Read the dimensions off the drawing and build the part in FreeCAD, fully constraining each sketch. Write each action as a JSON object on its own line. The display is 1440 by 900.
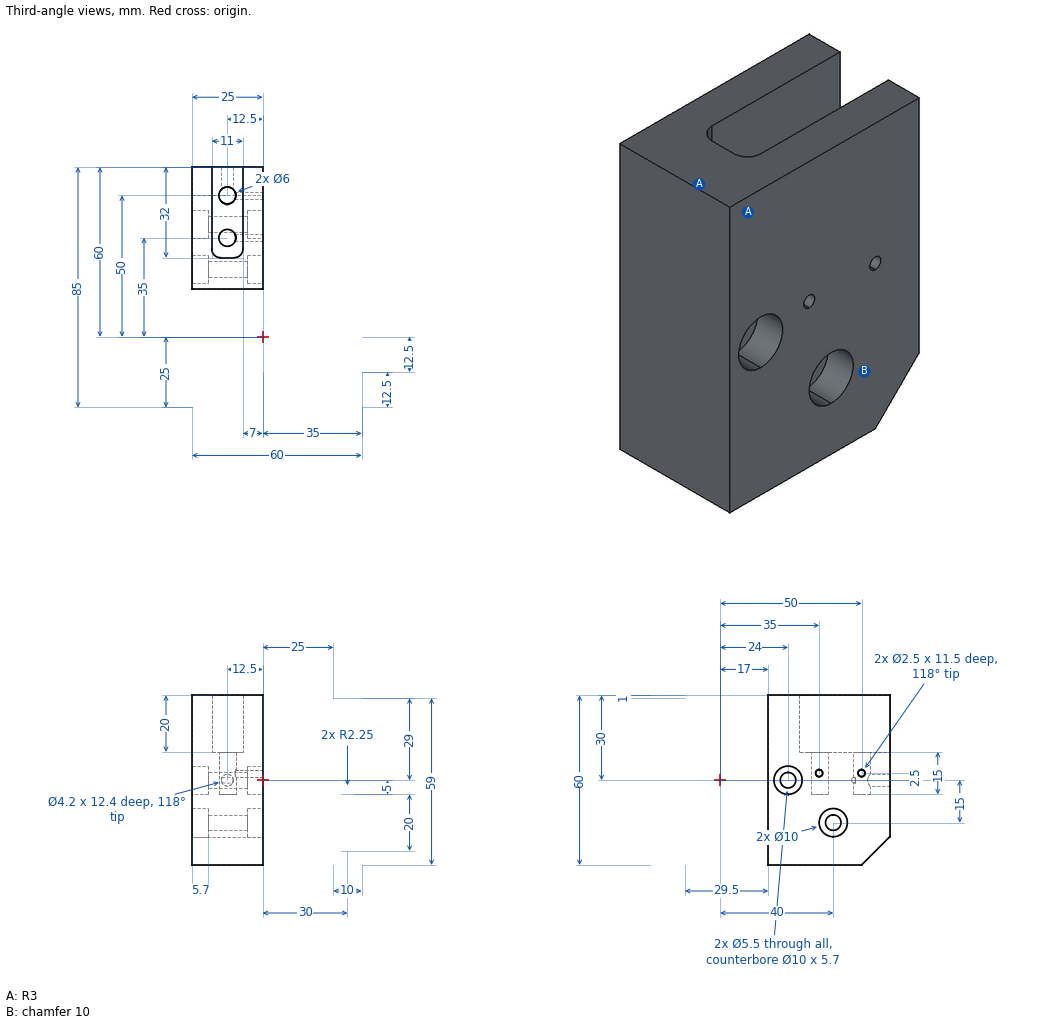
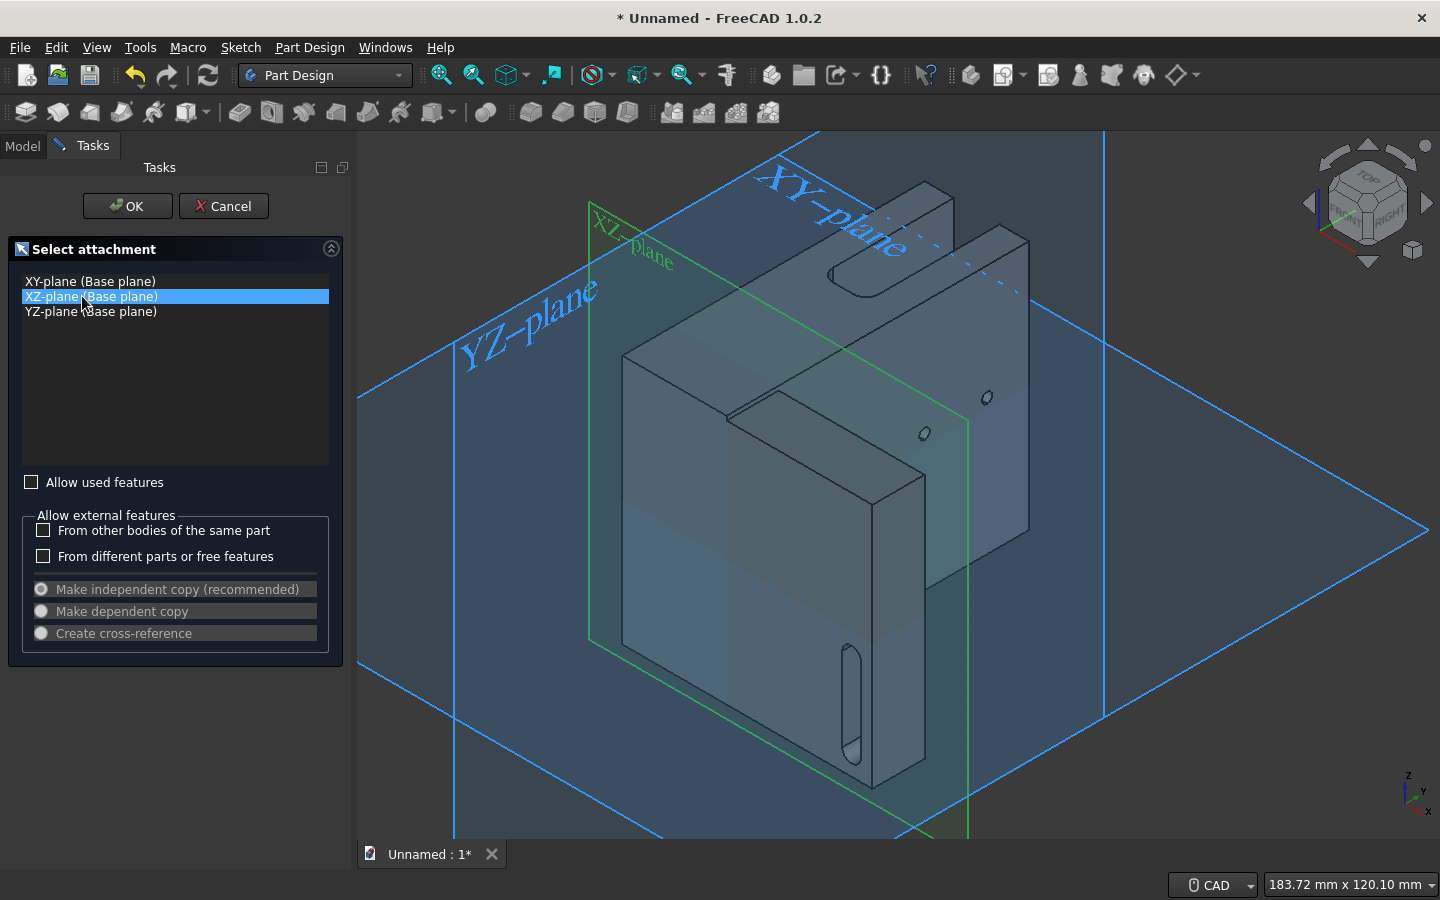
{"action": "left_click", "coordinate": [128, 206]}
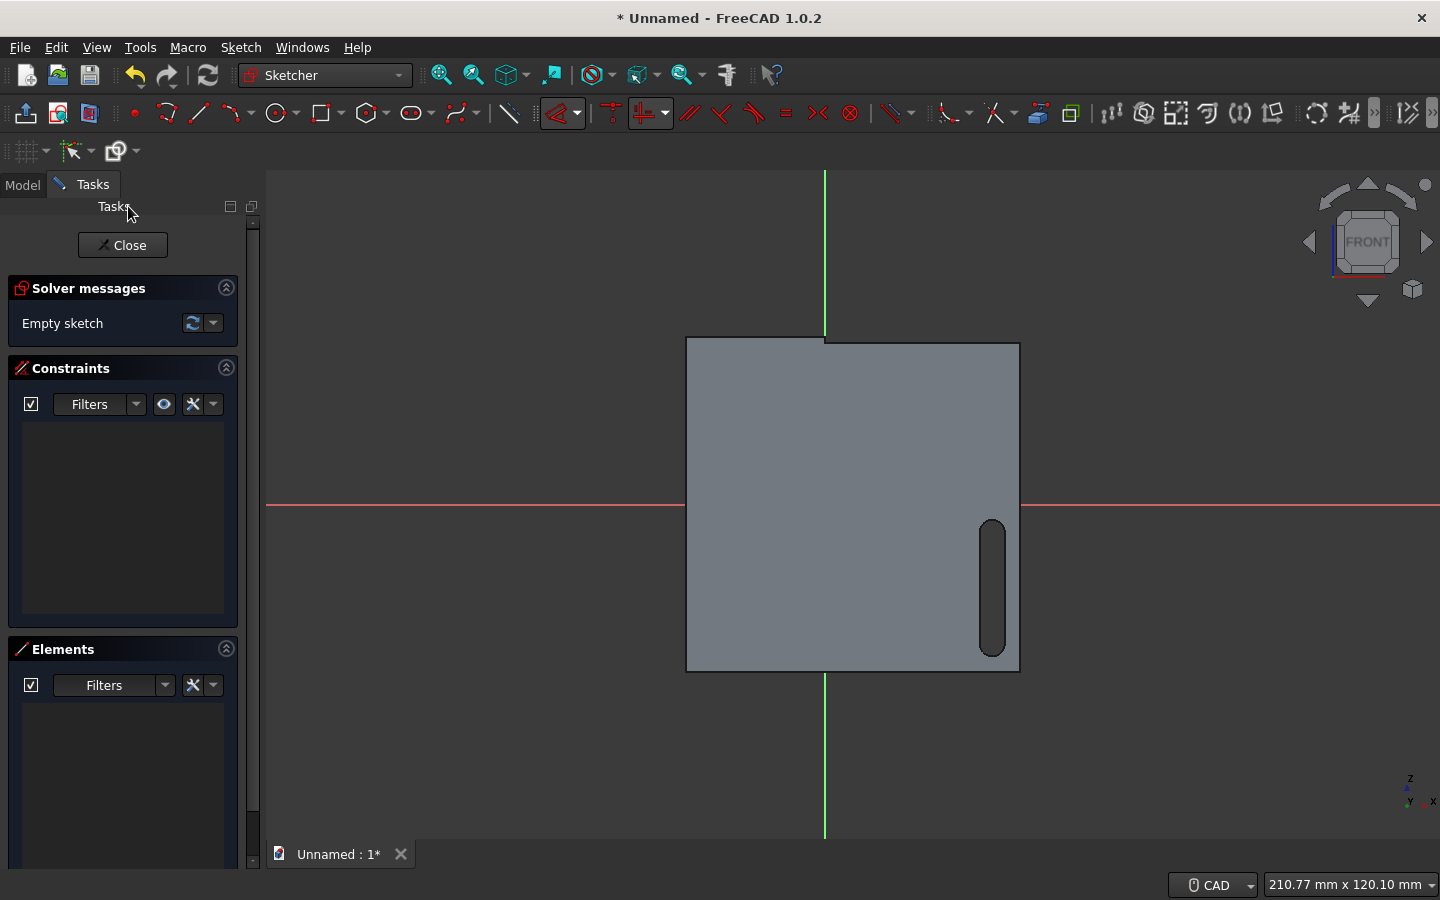
{"action": "left_click", "coordinate": [90, 114]}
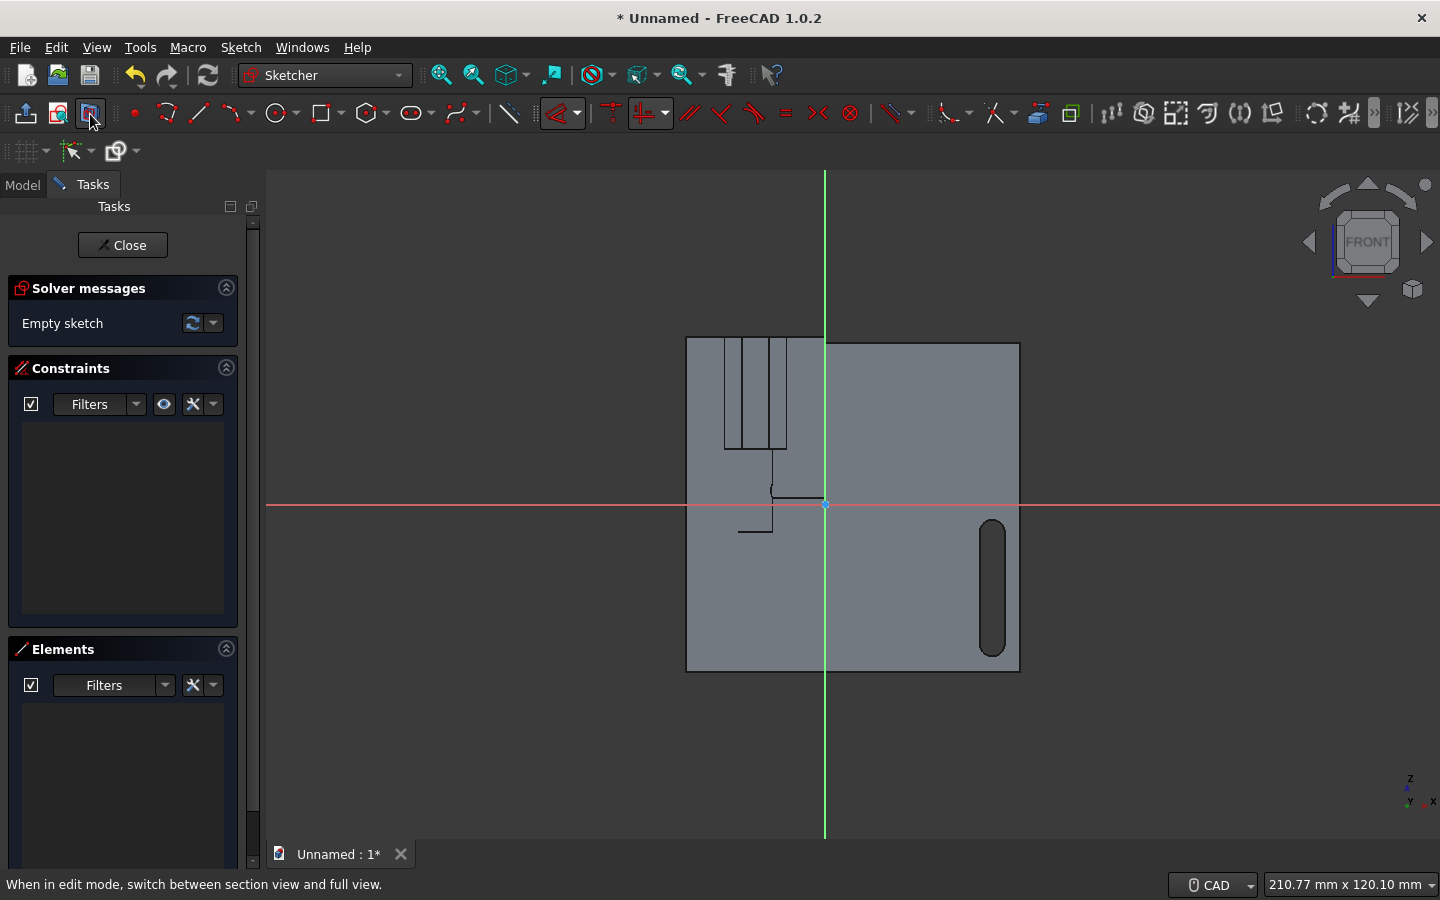
{"action": "left_click", "coordinate": [322, 114]}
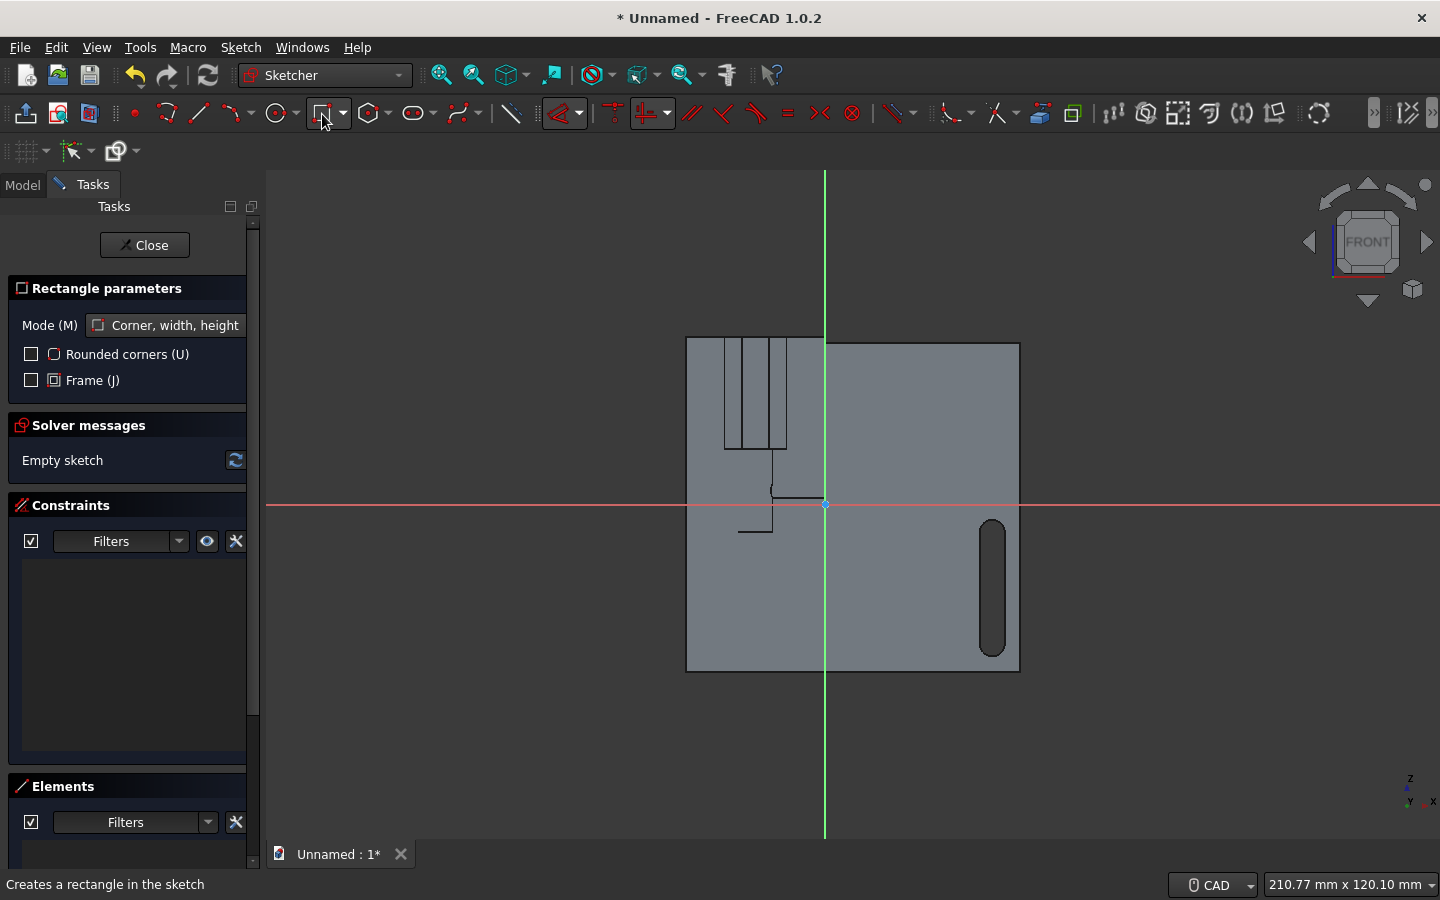
{"action": "left_click", "coordinate": [964, 343]}
{"action": "mouse_move", "coordinate": [1020, 672]}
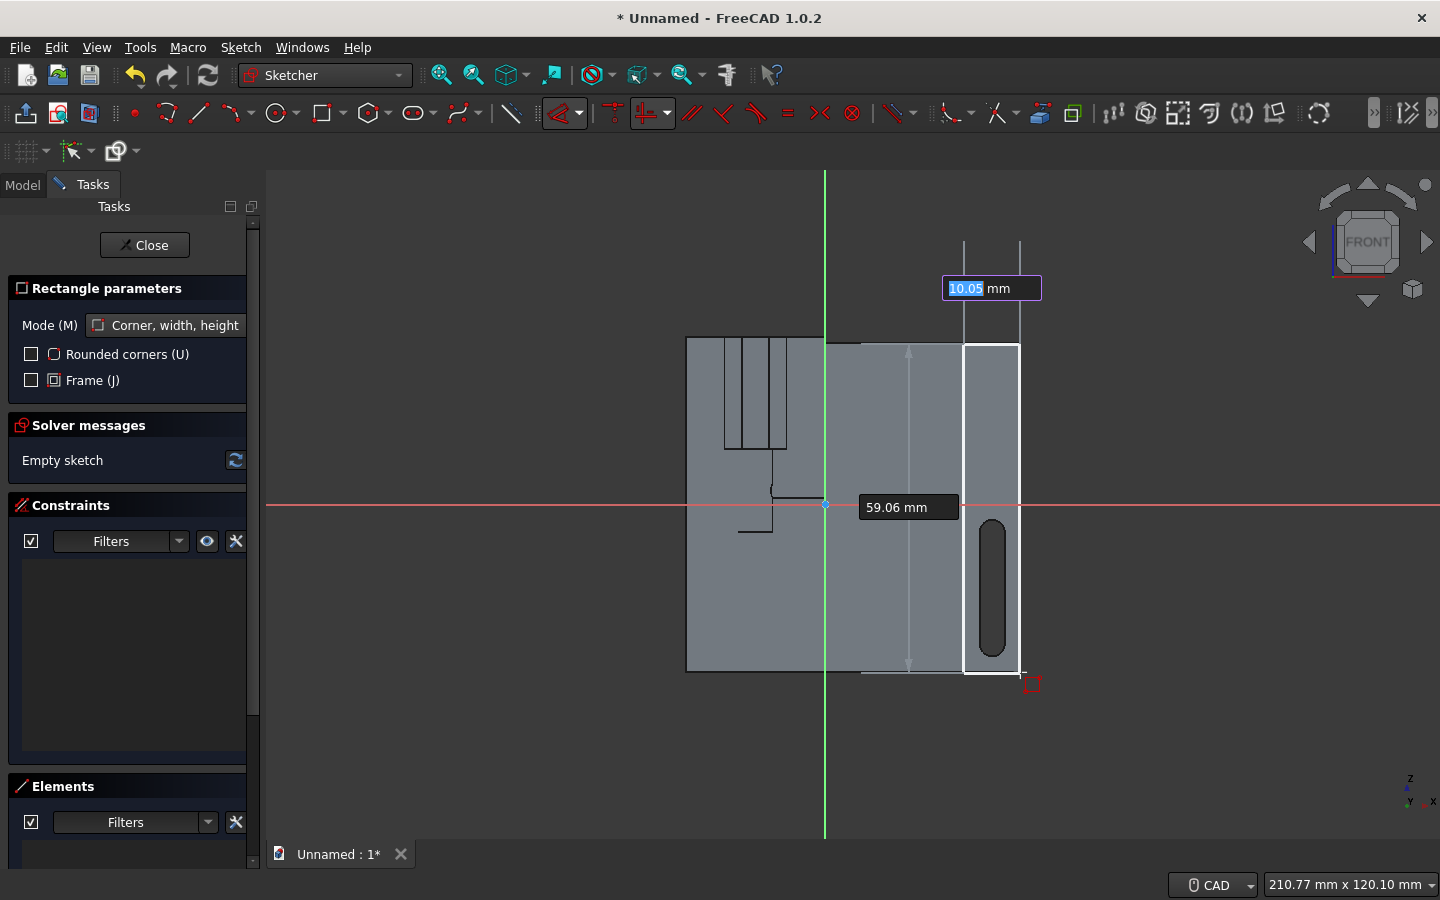
{"action": "type", "text": "10"}
{"action": "key", "text": "Tab"}
{"action": "type", "text": "59"}
{"action": "key", "text": "Return"}
{"action": "key", "text": "Escape"}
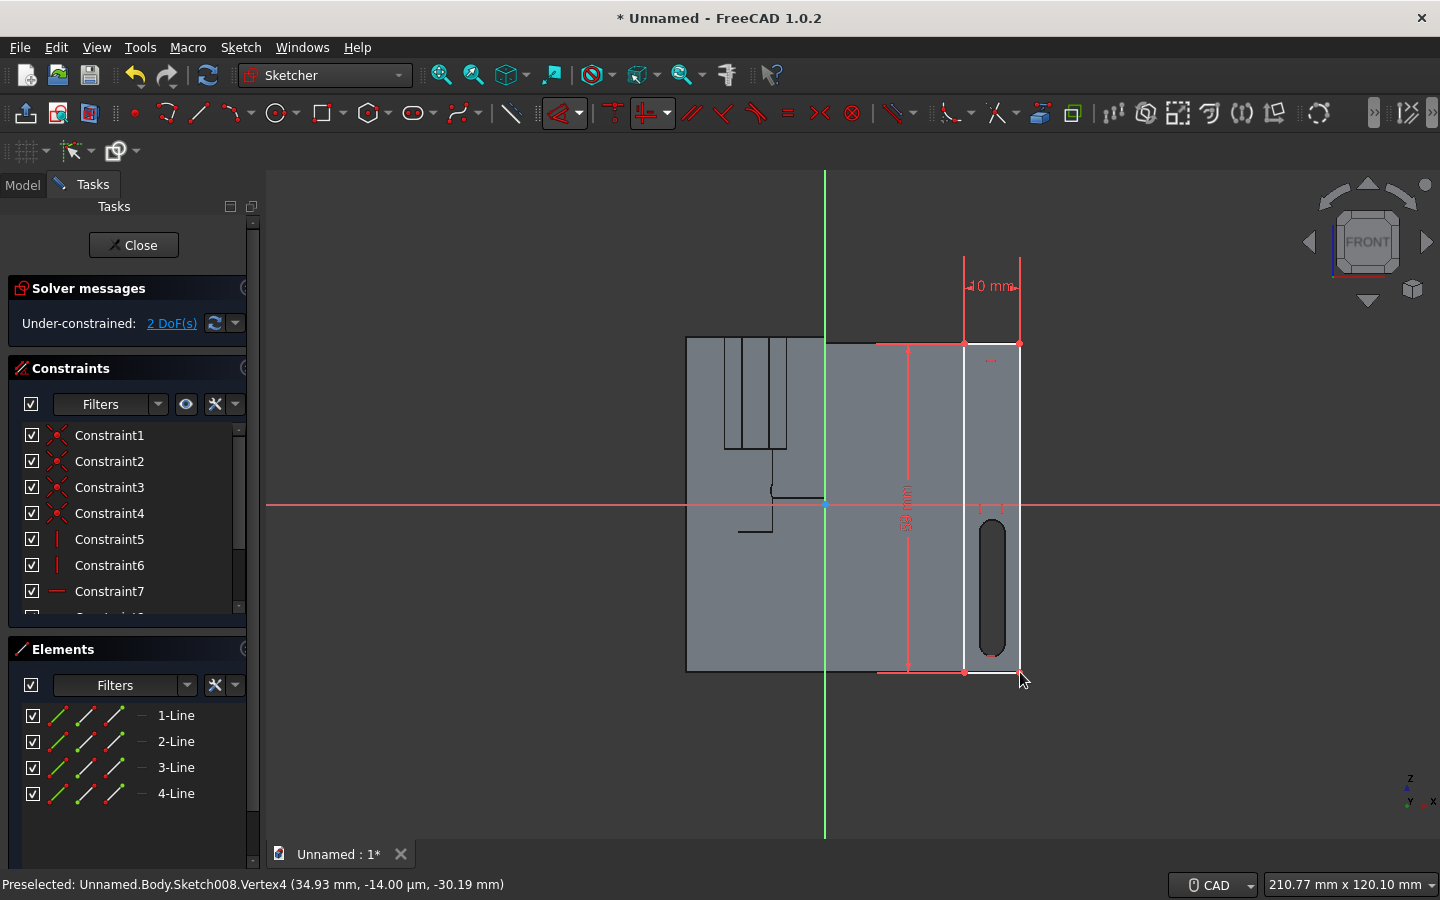
{"action": "left_click", "coordinate": [964, 344]}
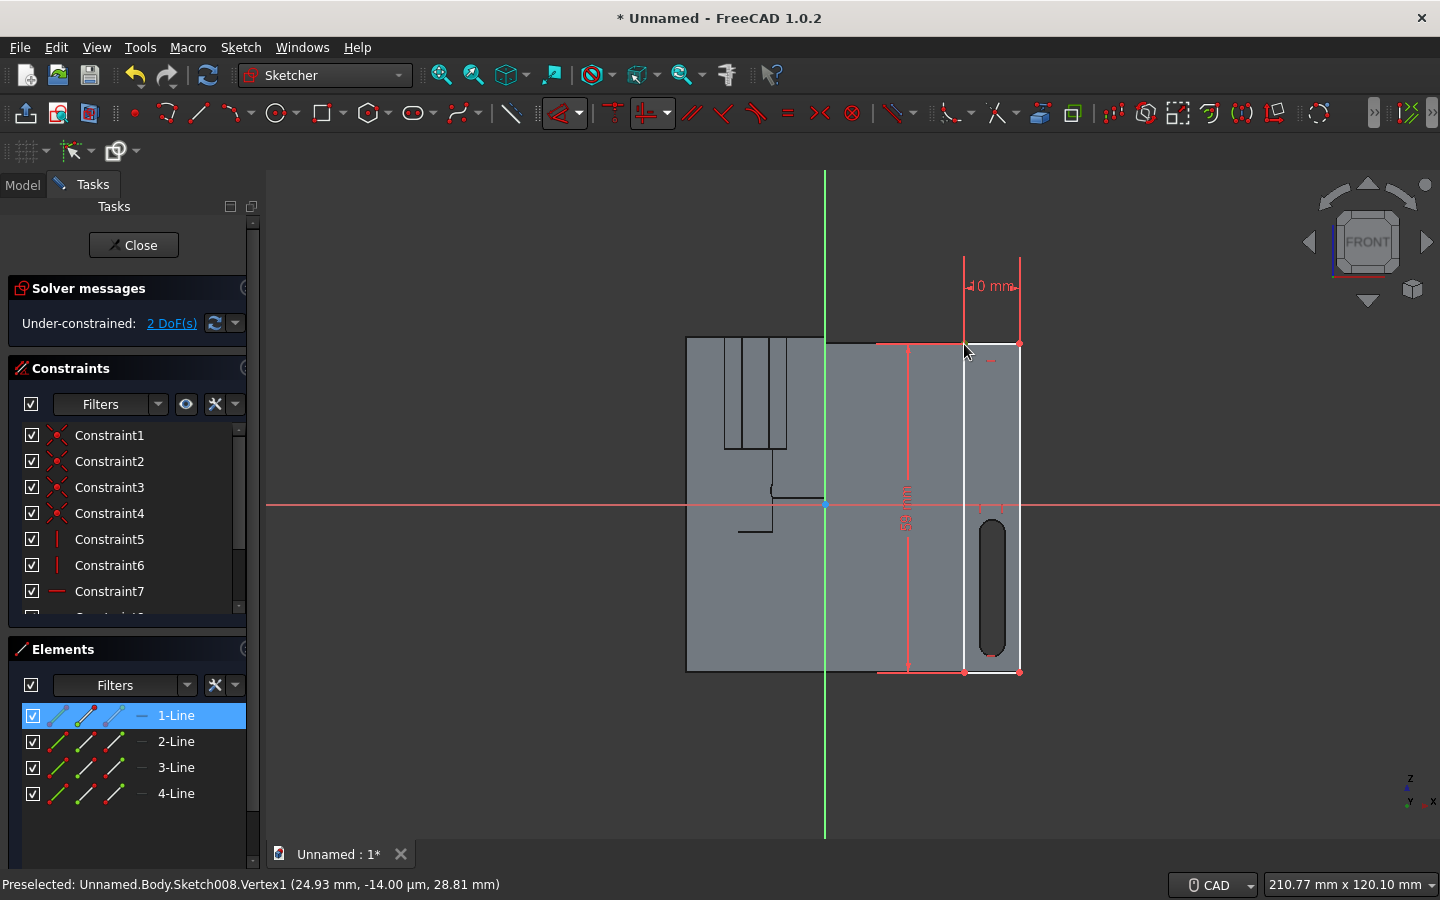
{"action": "left_click", "coordinate": [582, 114]}